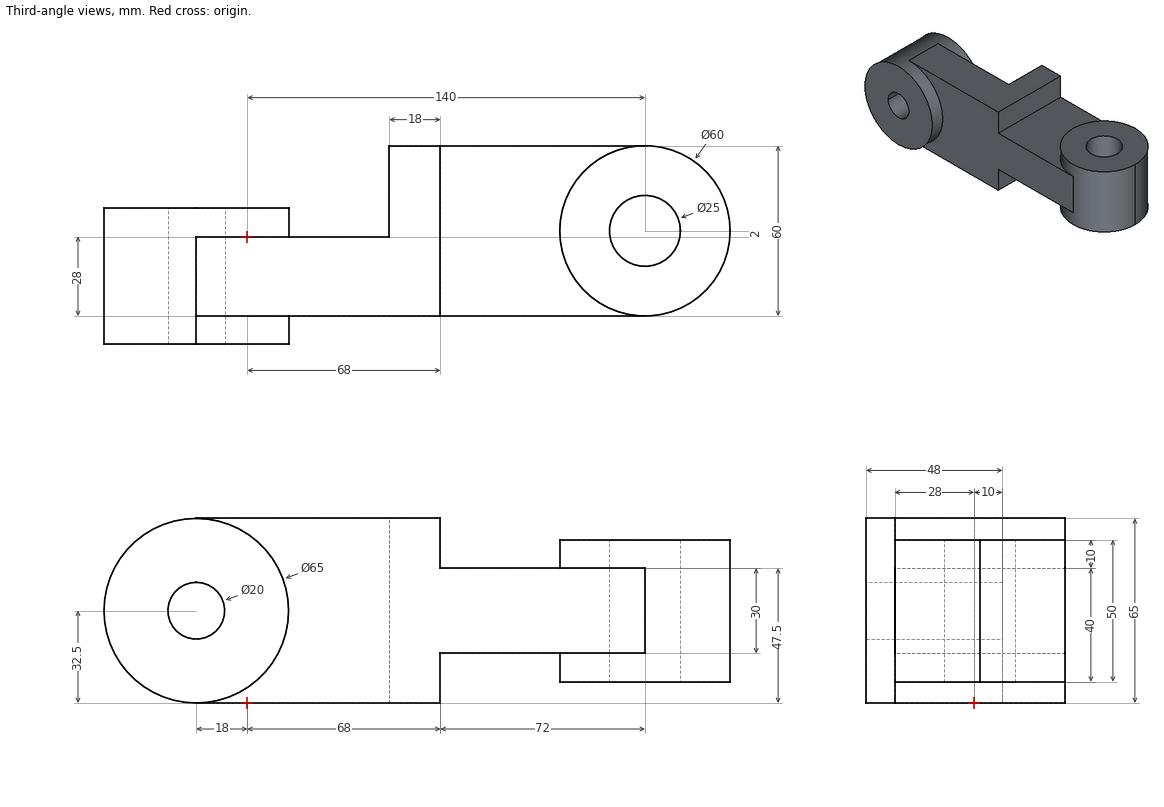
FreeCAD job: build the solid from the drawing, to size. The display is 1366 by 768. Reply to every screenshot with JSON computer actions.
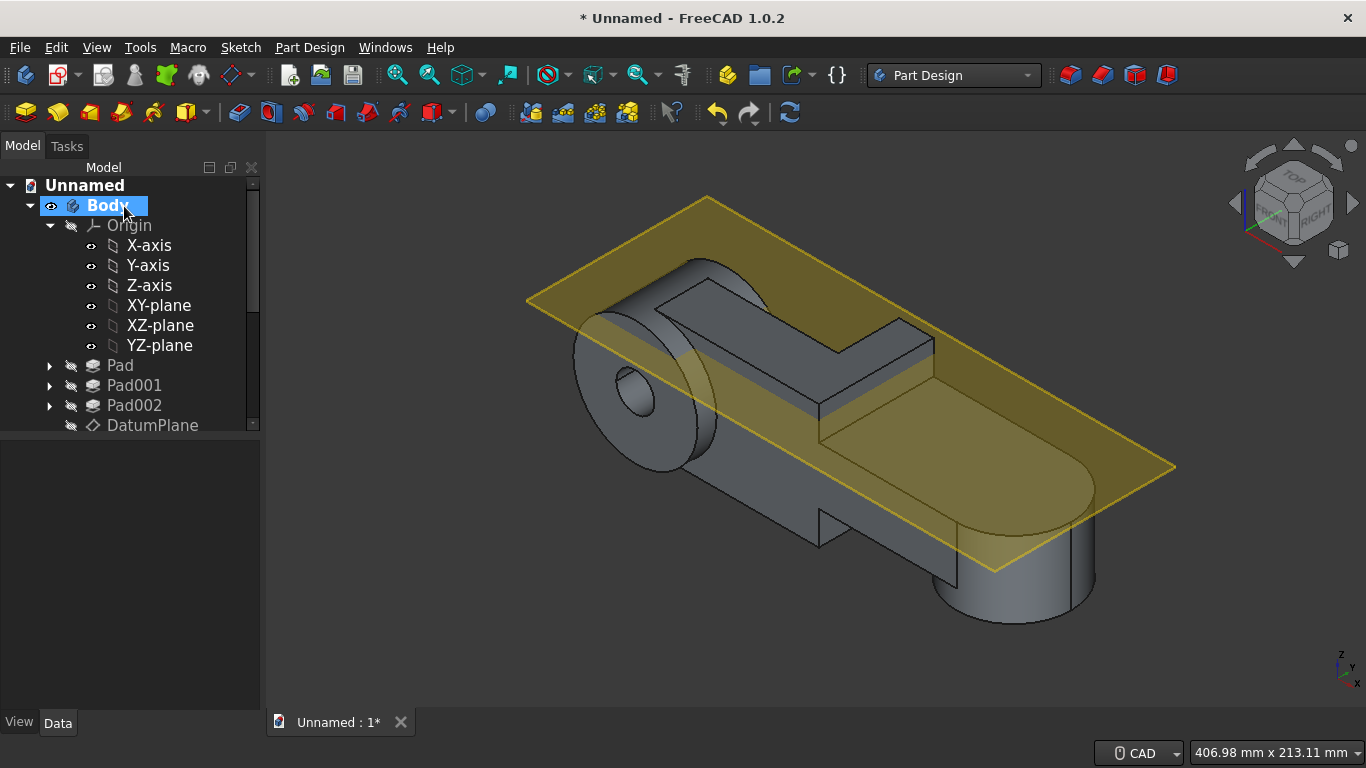
{"action": "scroll", "coordinate": [100, 301], "scroll_direction": "down", "scroll_amount": 3}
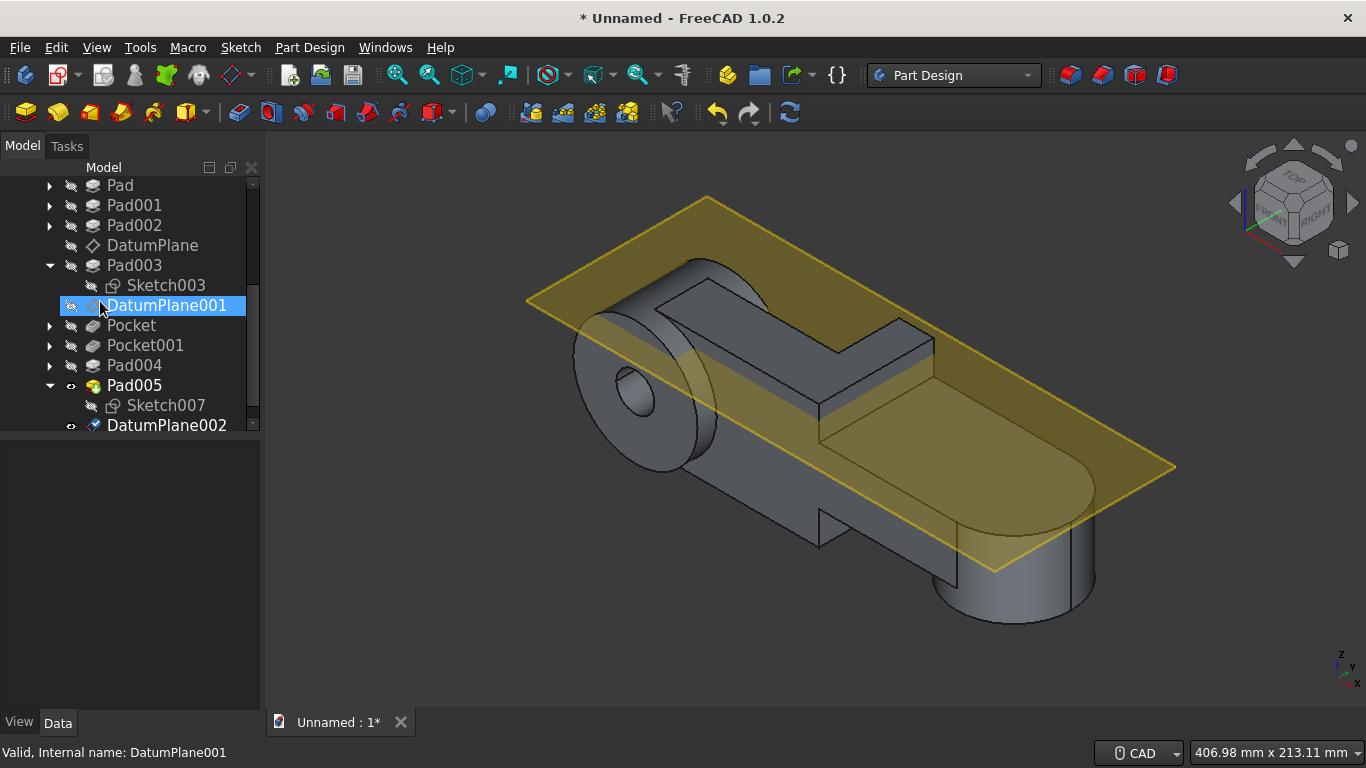
{"action": "left_click", "coordinate": [116, 426]}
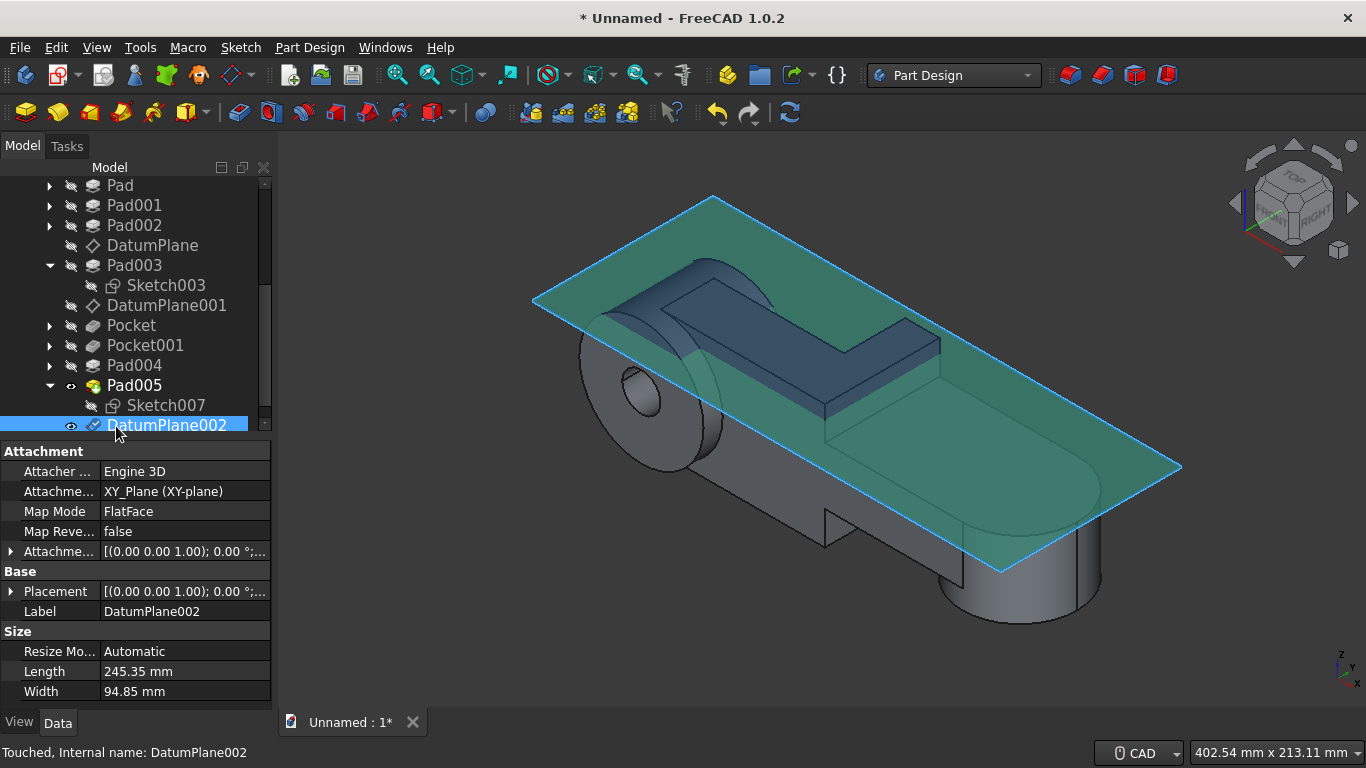
{"action": "left_click", "coordinate": [58, 76]}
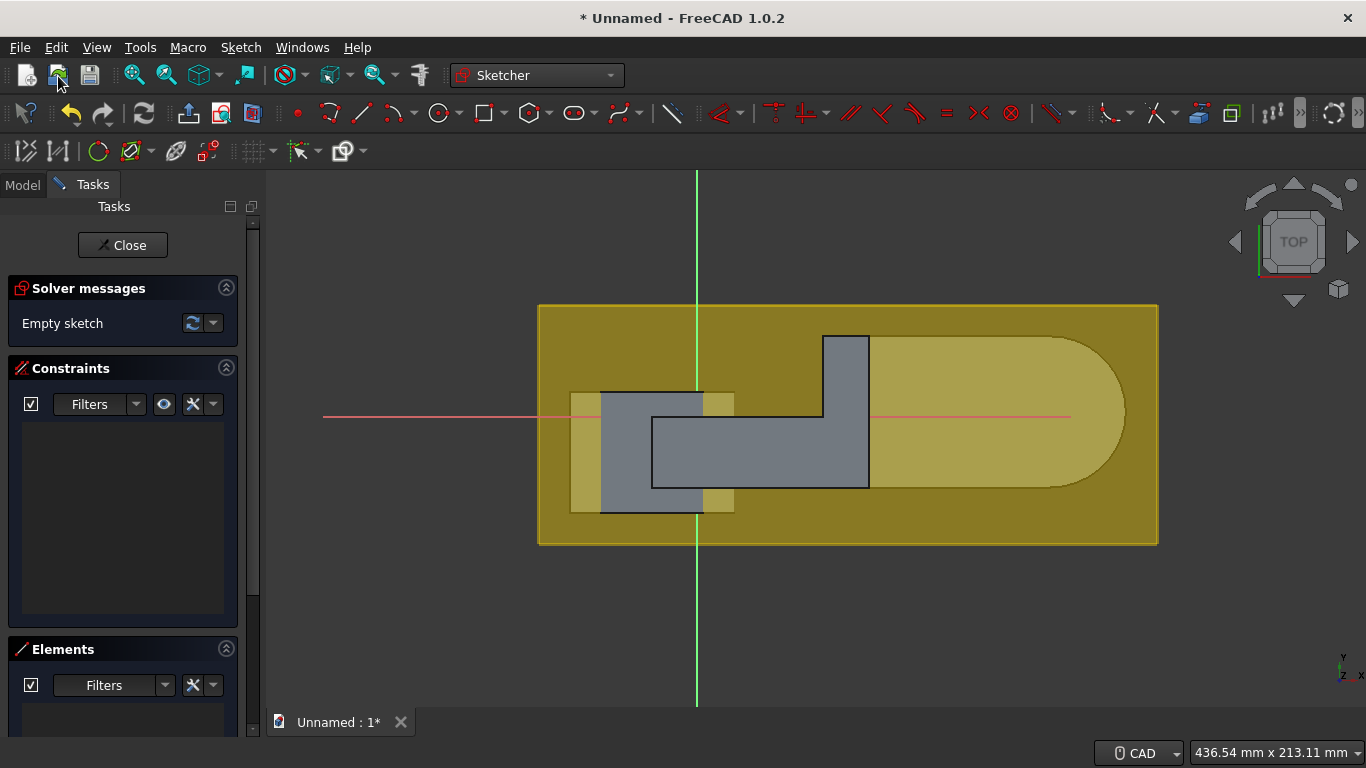
{"action": "key", "text": "q s"}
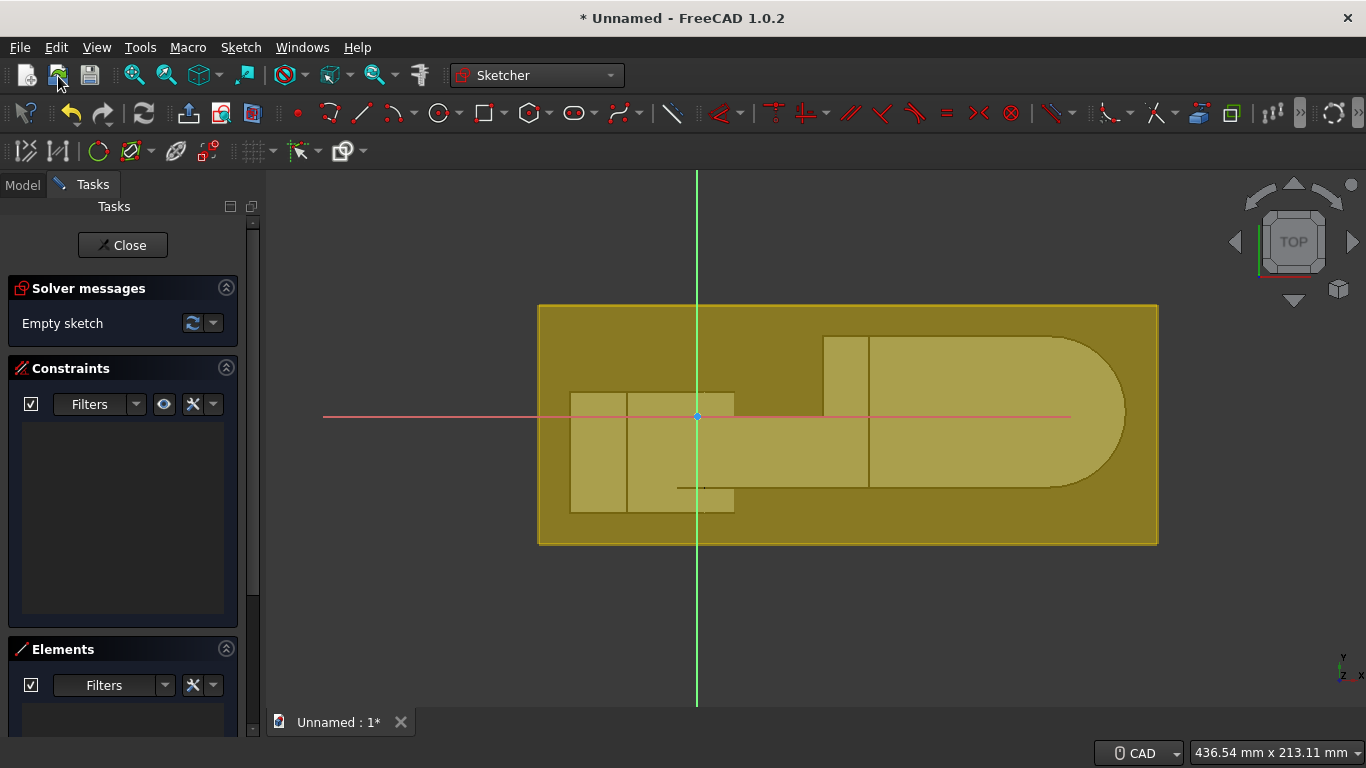
{"action": "scroll", "coordinate": [1201, 390], "scroll_direction": "up", "scroll_amount": 4}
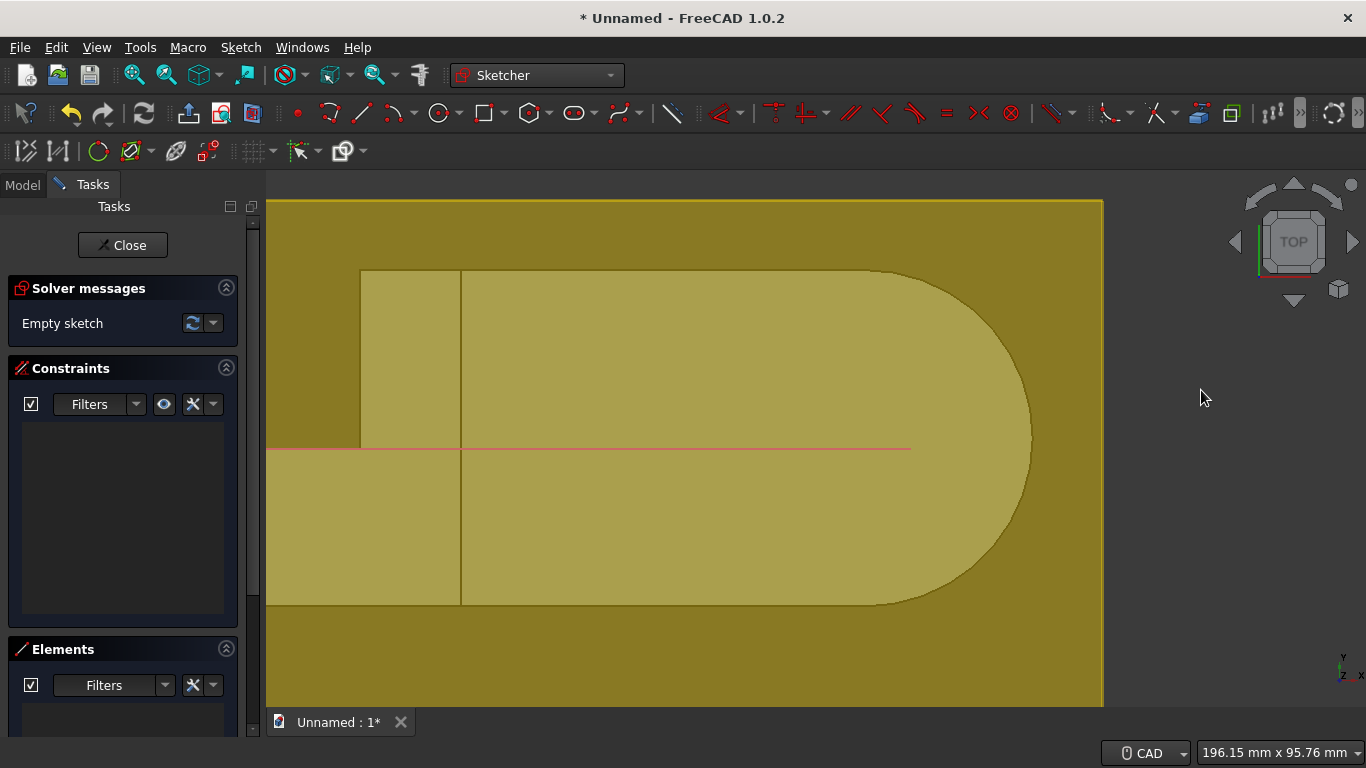
{"action": "key", "text": "g c"}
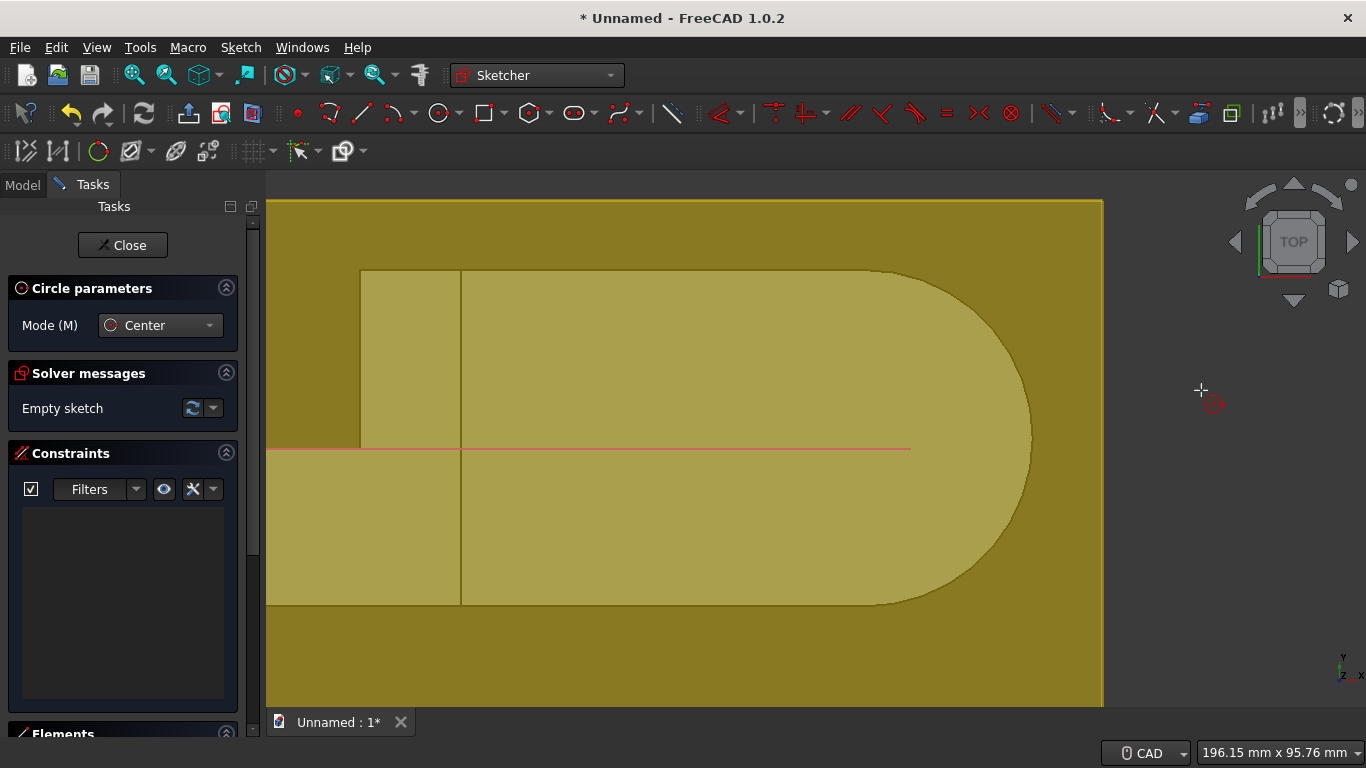
{"action": "scroll", "coordinate": [864, 438], "scroll_direction": "up", "scroll_amount": 2}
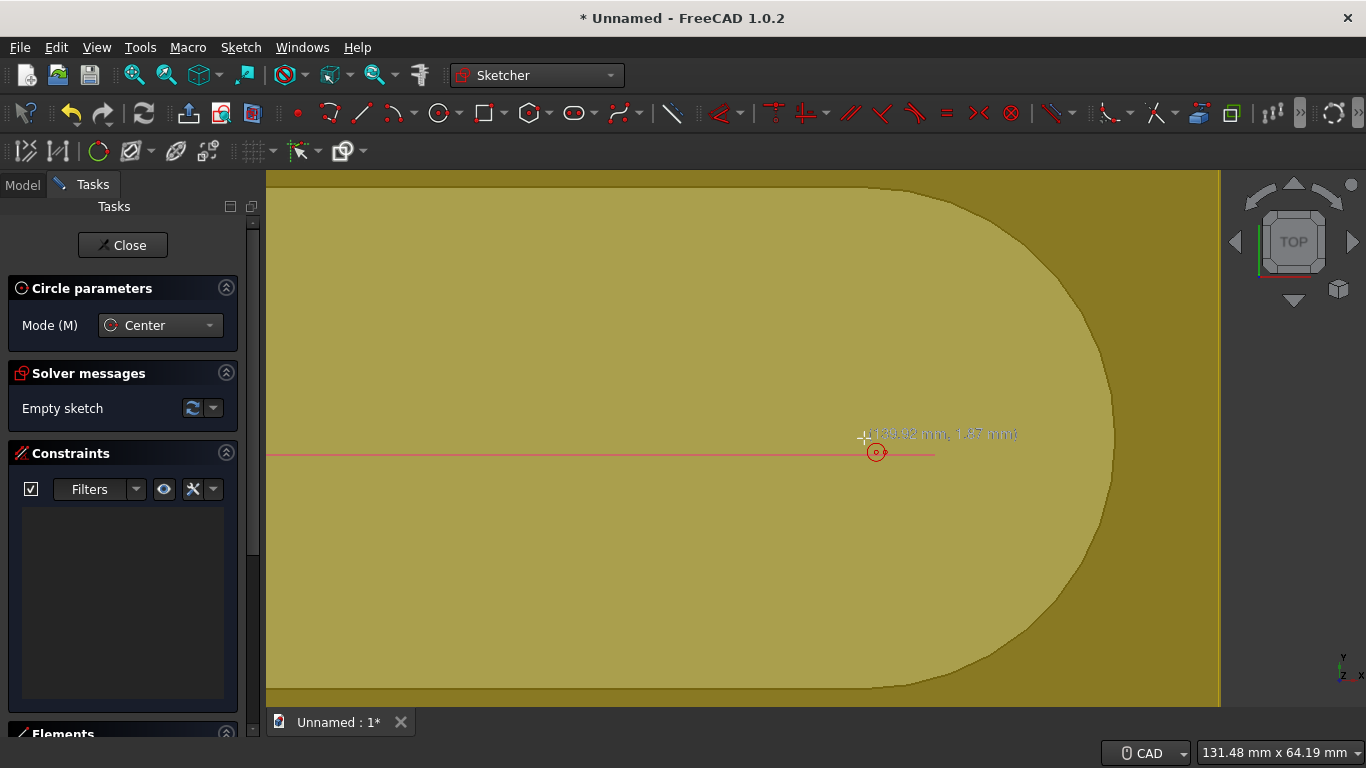
{"action": "left_click", "coordinate": [864, 438]}
{"action": "left_click", "coordinate": [1042, 261]}
{"action": "key", "text": "Escape"}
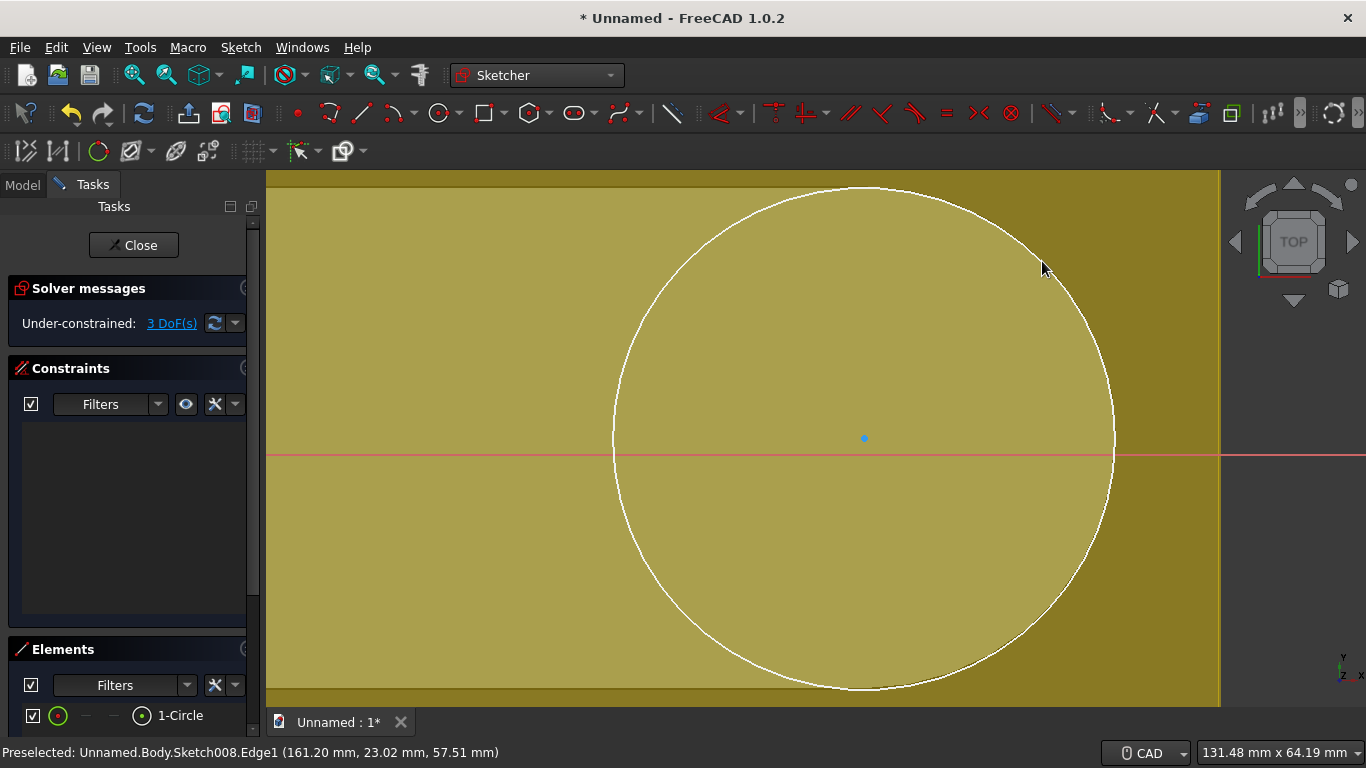
{"action": "key", "text": "d"}